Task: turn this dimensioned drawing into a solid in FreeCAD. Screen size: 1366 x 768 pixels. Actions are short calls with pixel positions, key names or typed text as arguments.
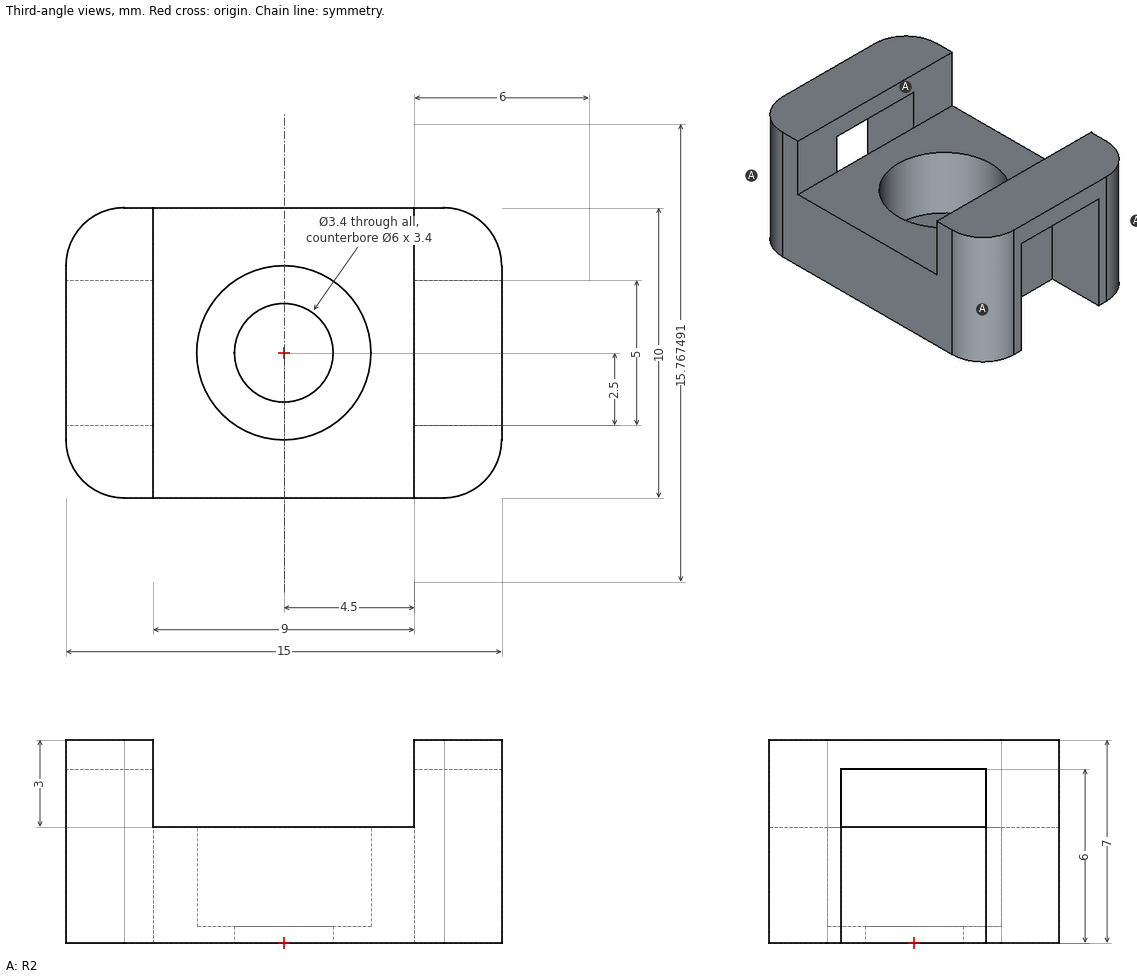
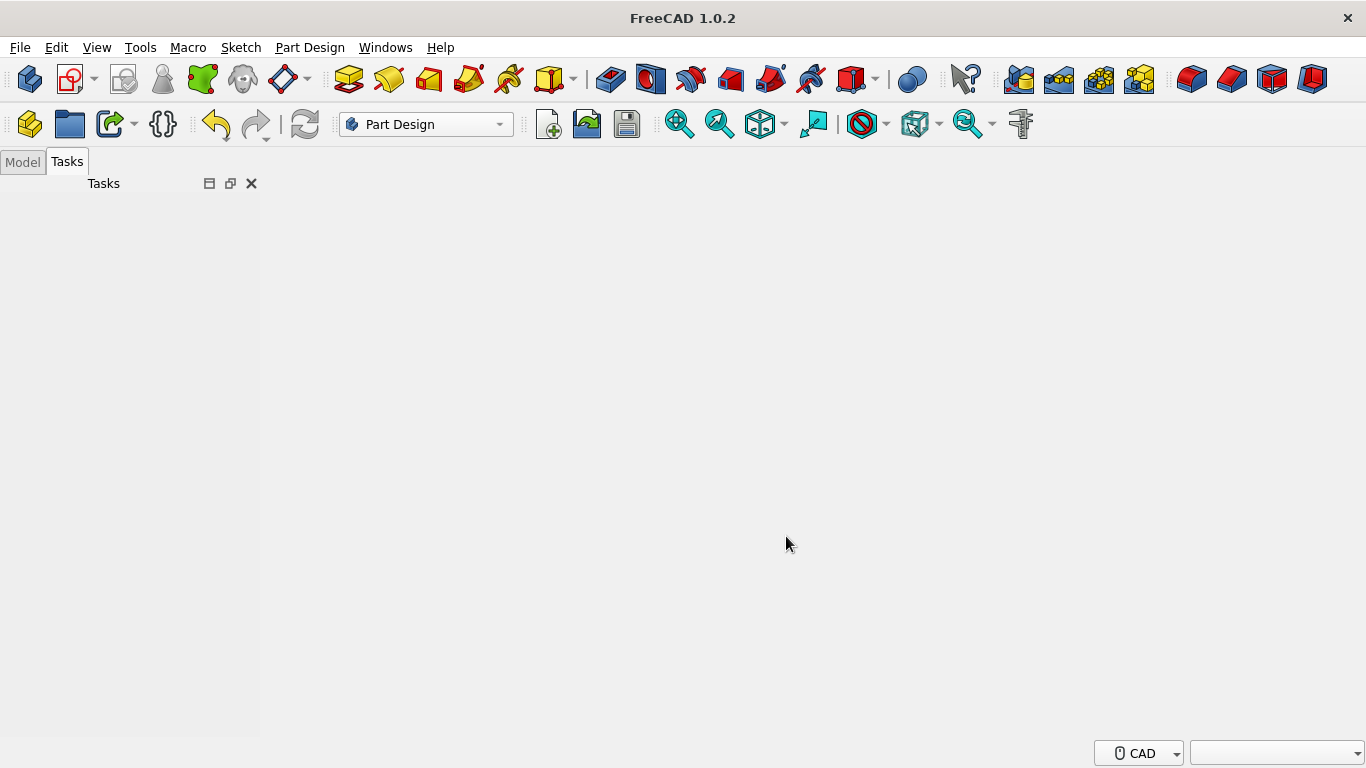
click(548, 124)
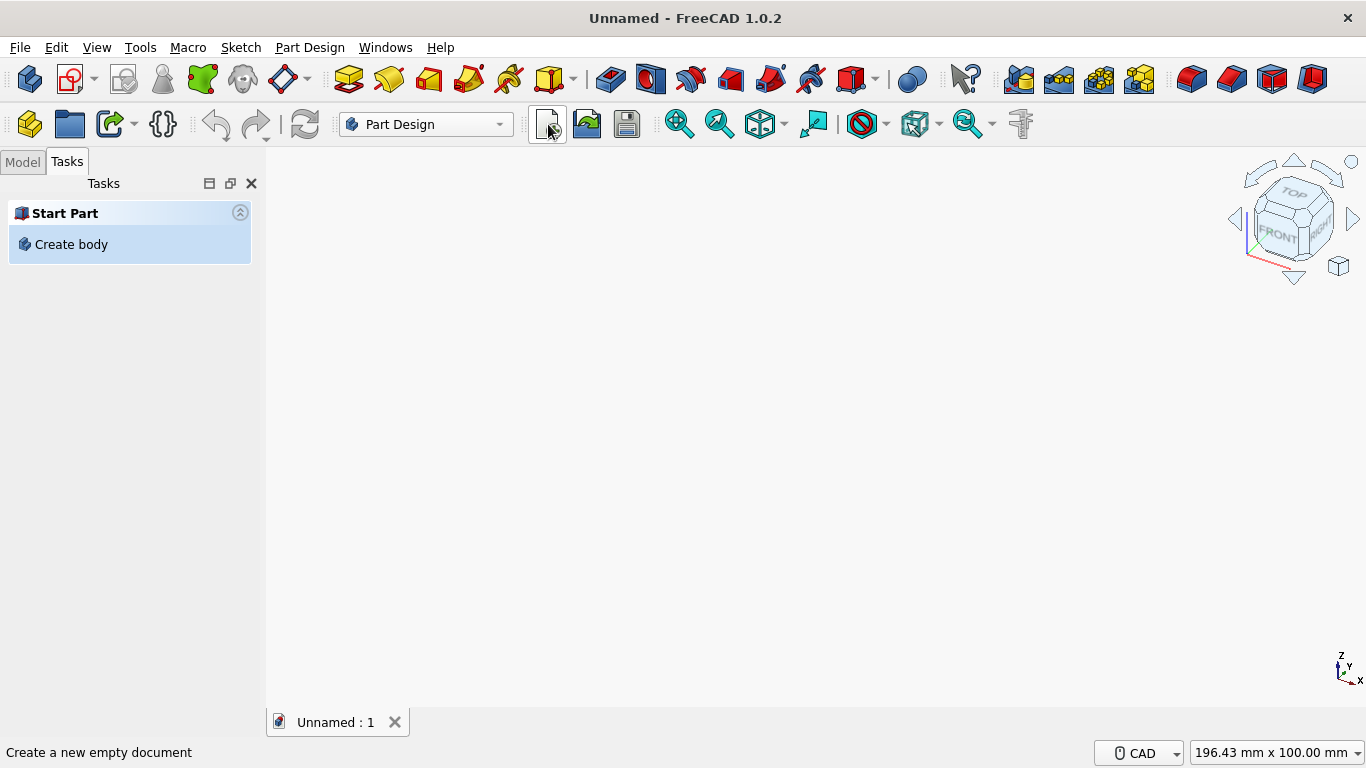
click(70, 80)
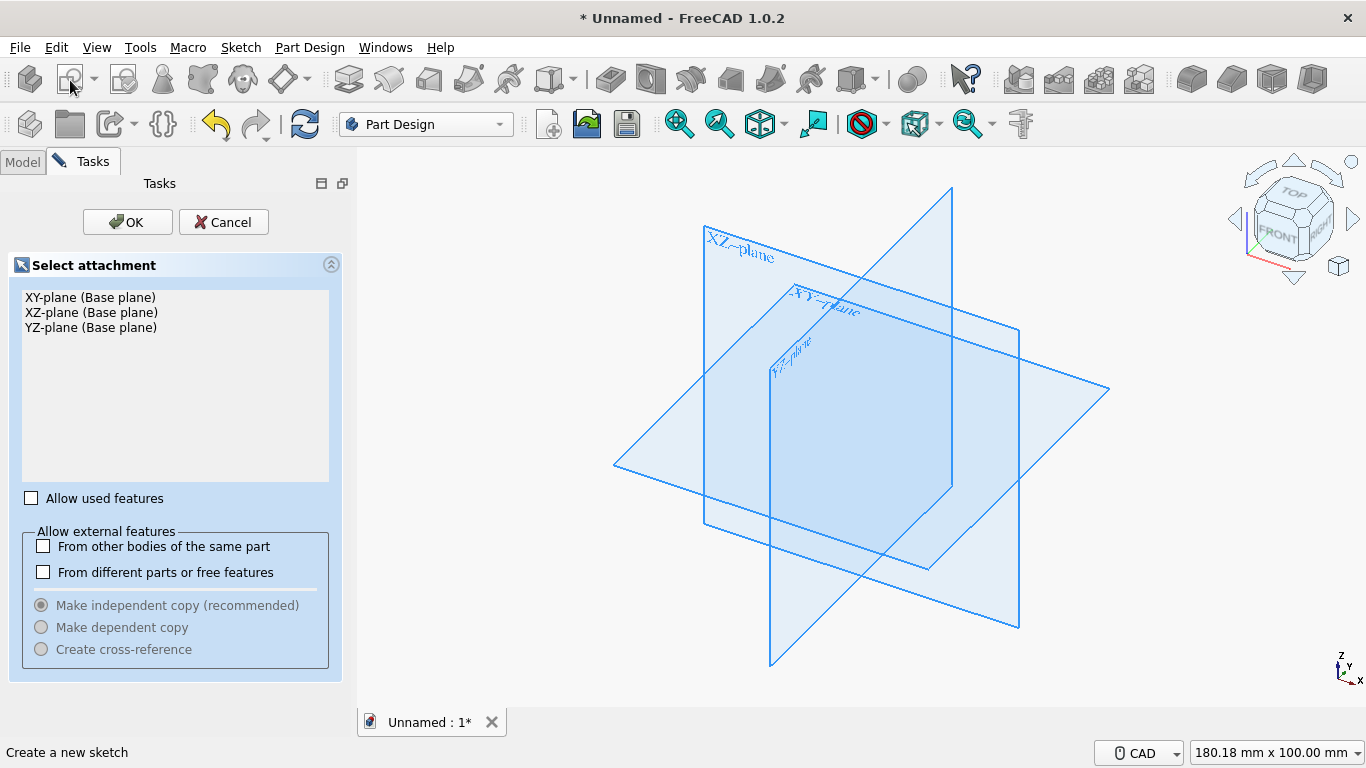
click(82, 298)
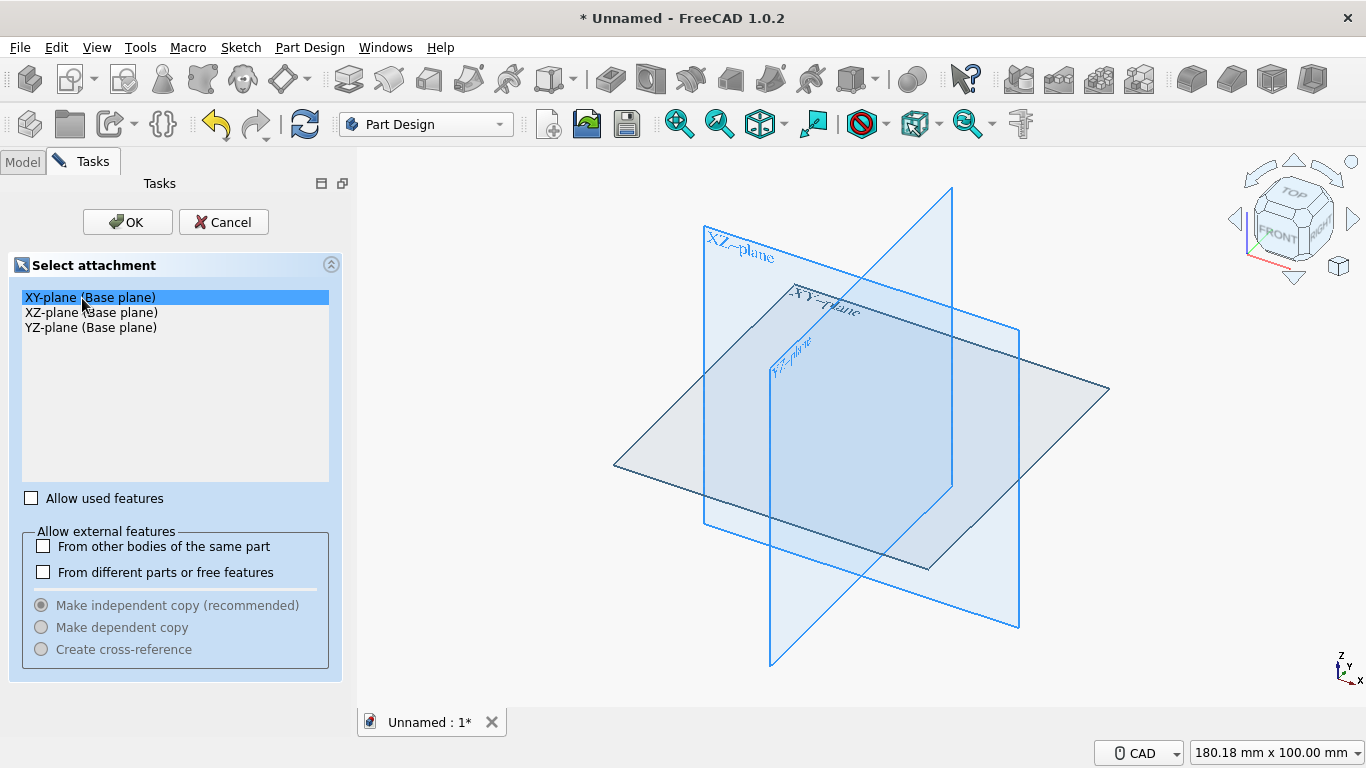
click(128, 222)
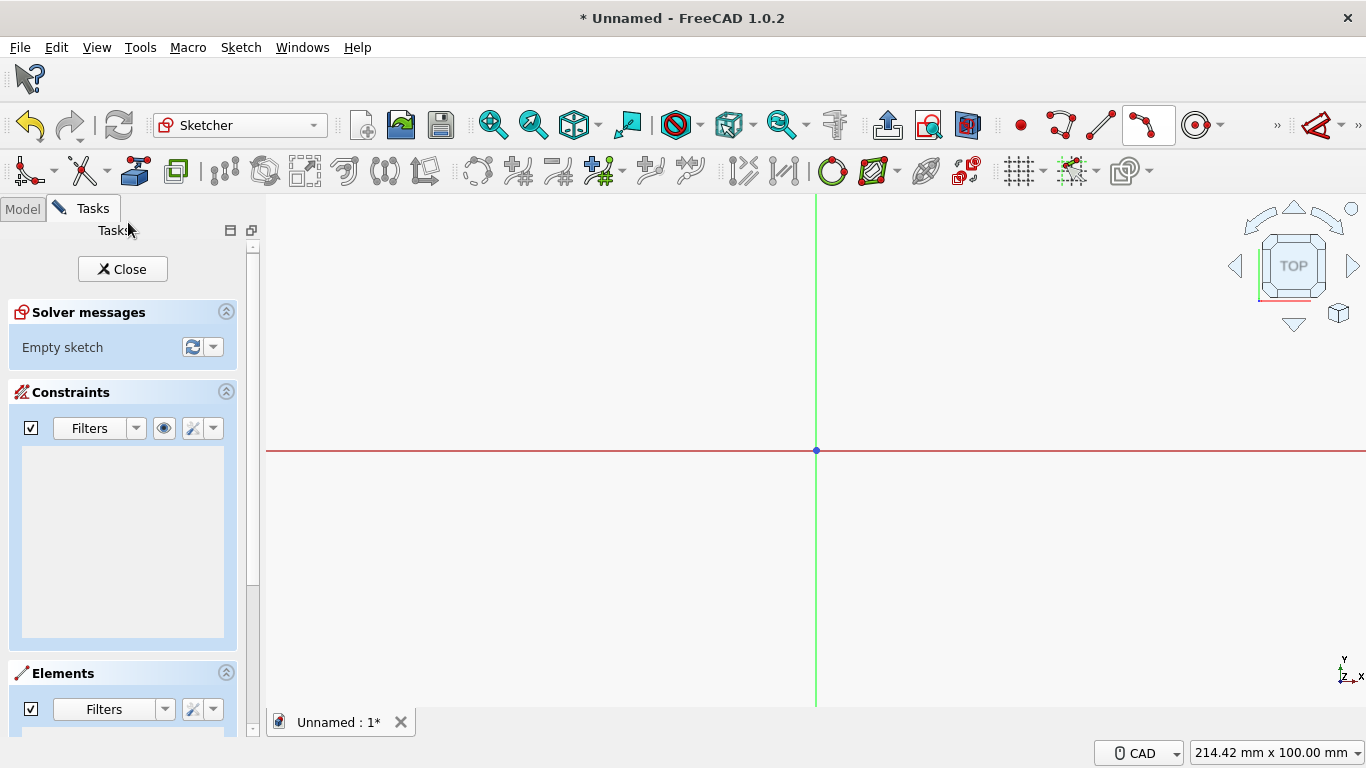
scroll(830, 451, up, 9)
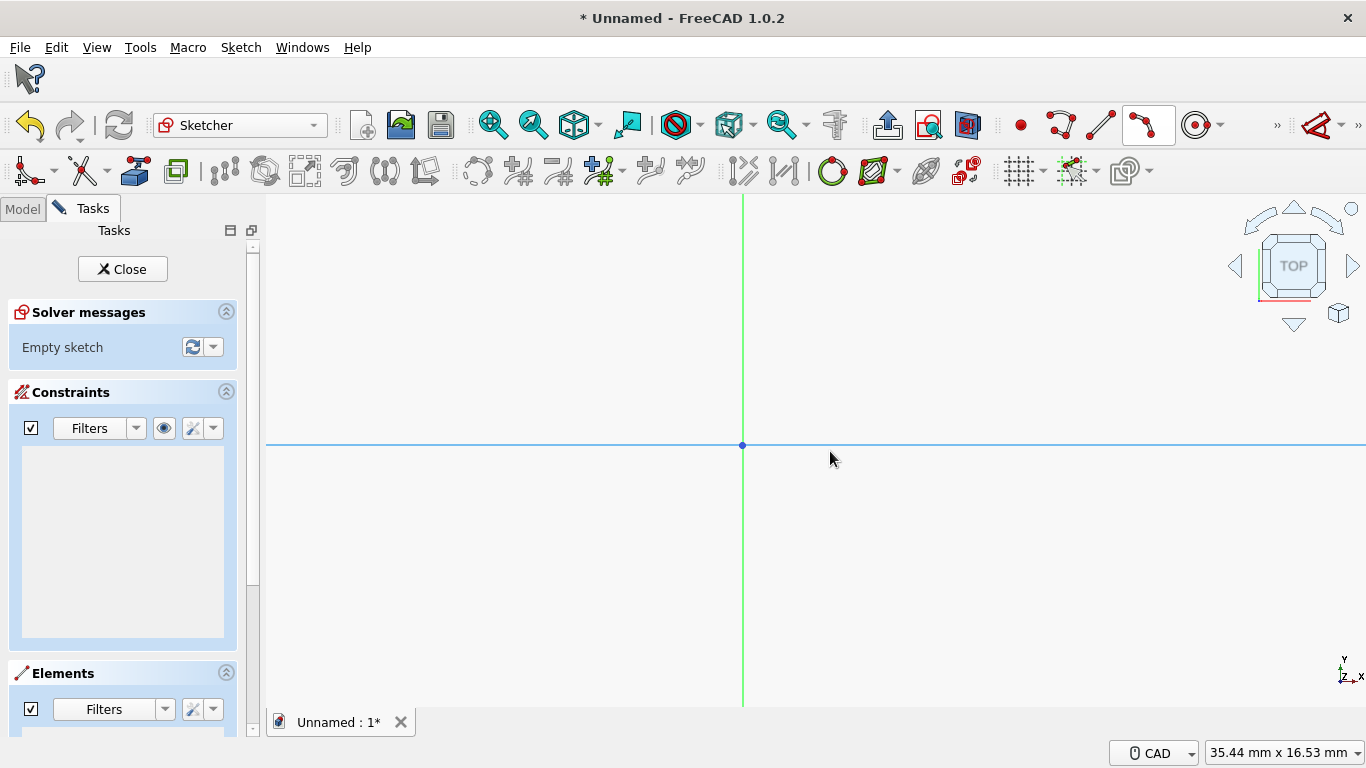
key(g)
key(v)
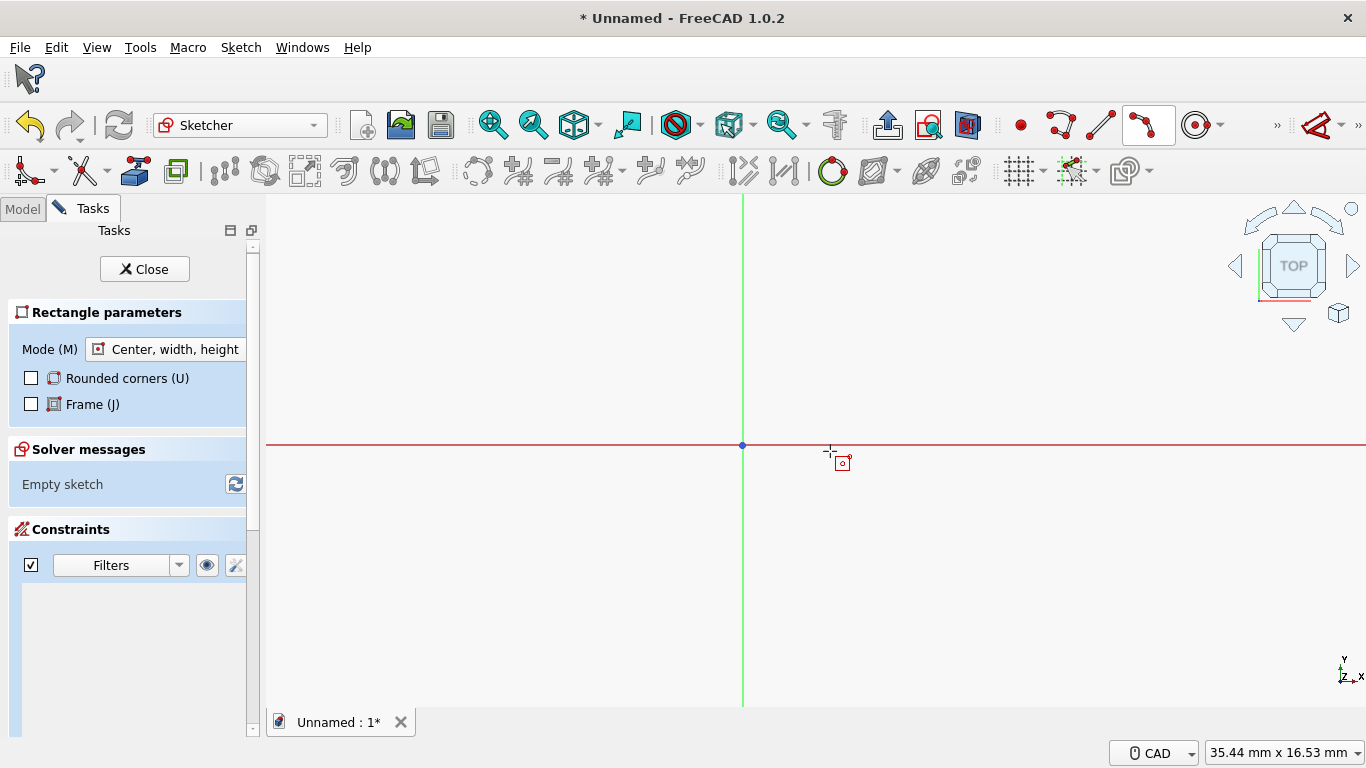
click(743, 445)
click(975, 290)
key(Escape)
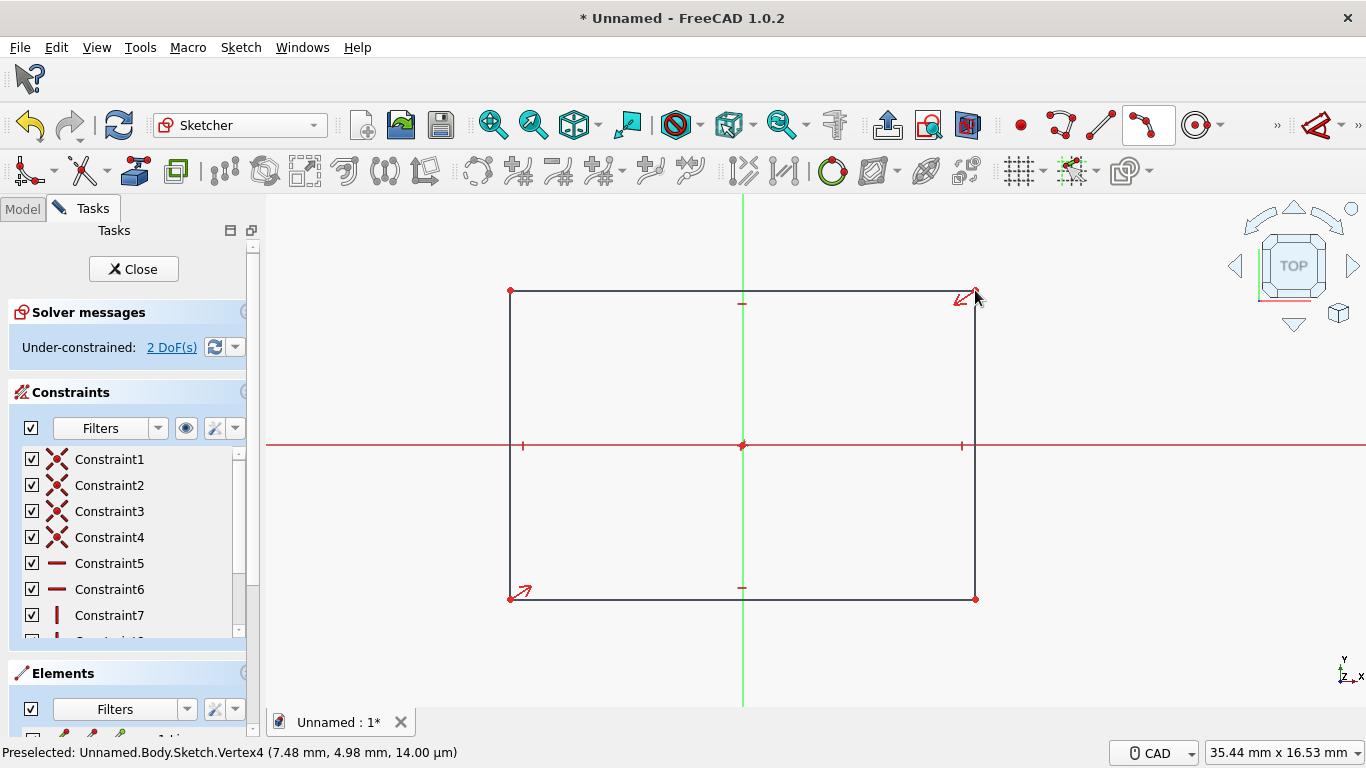
click(650, 600)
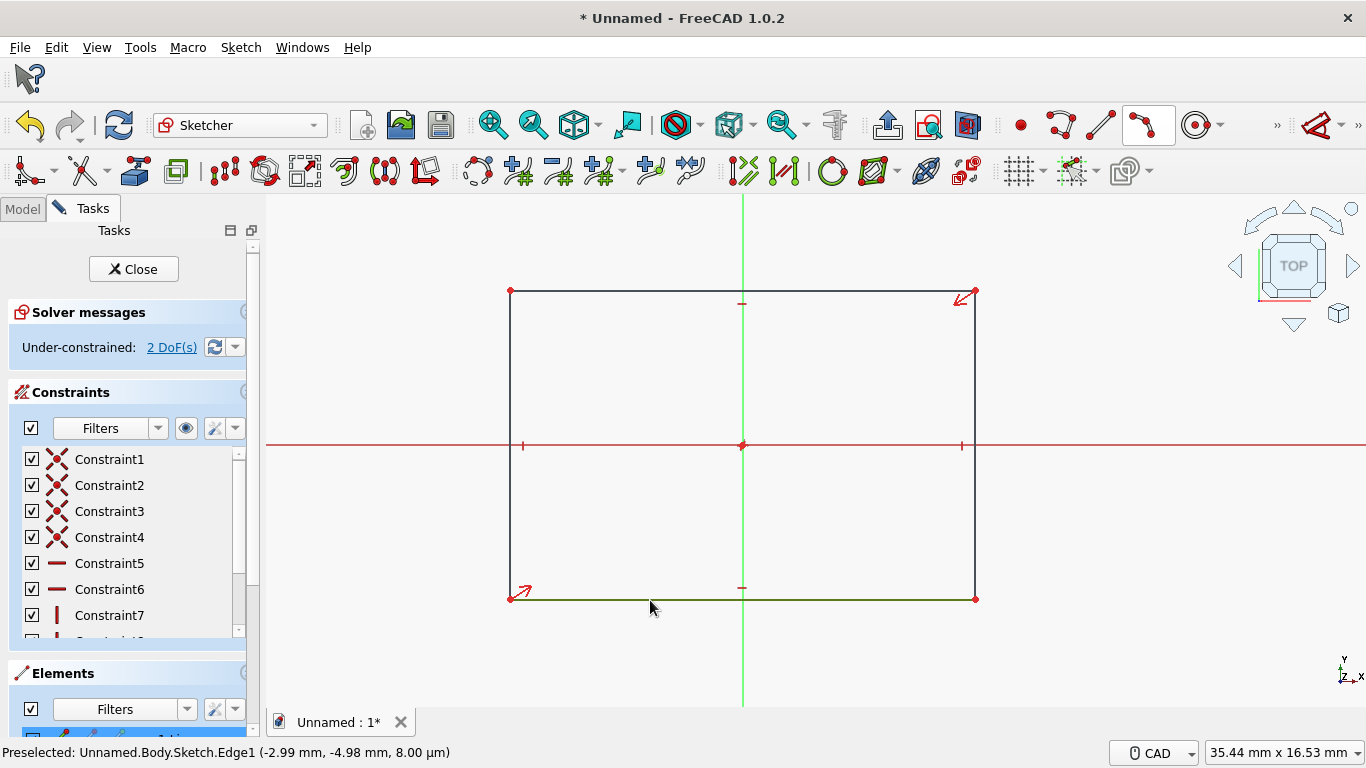
key(l)